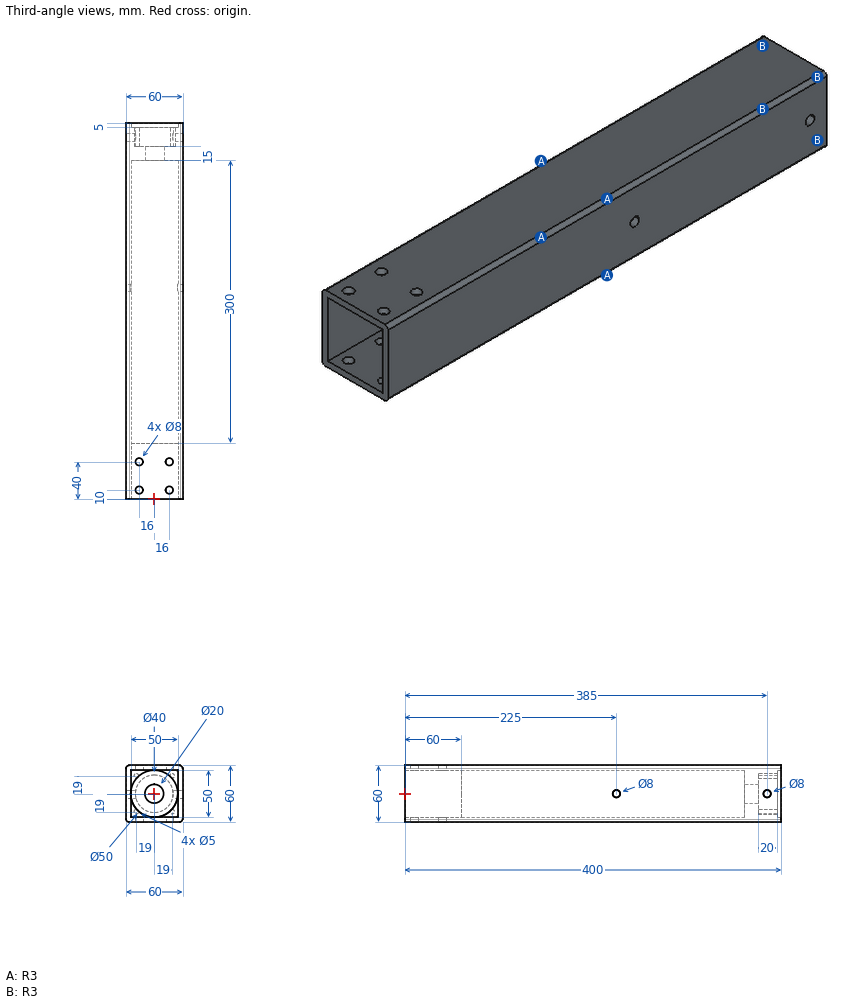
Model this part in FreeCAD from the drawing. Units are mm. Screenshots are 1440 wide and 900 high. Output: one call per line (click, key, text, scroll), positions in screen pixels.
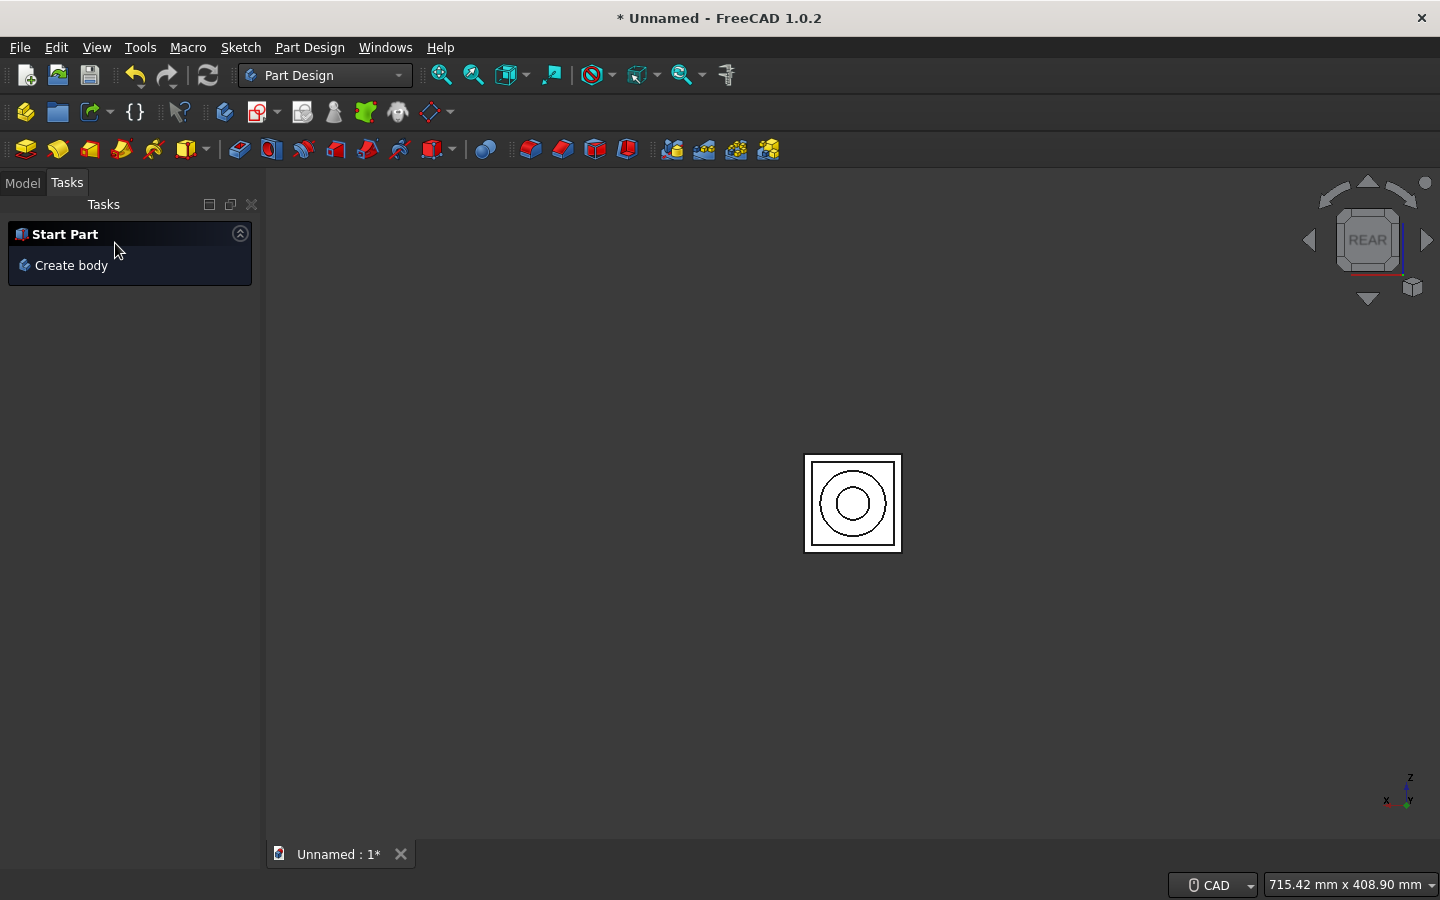
click(442, 76)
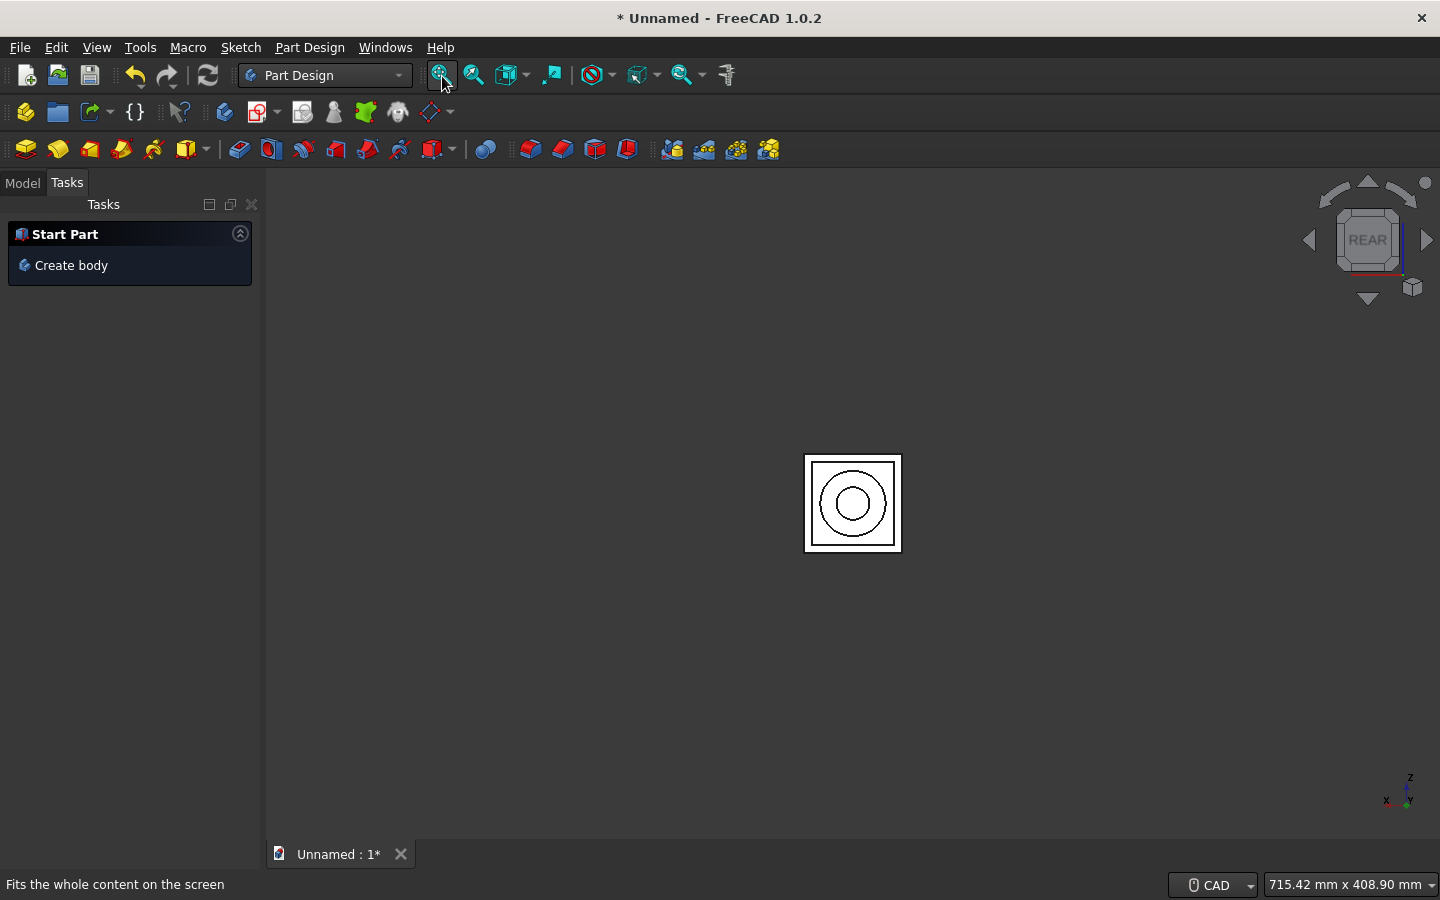
key(0)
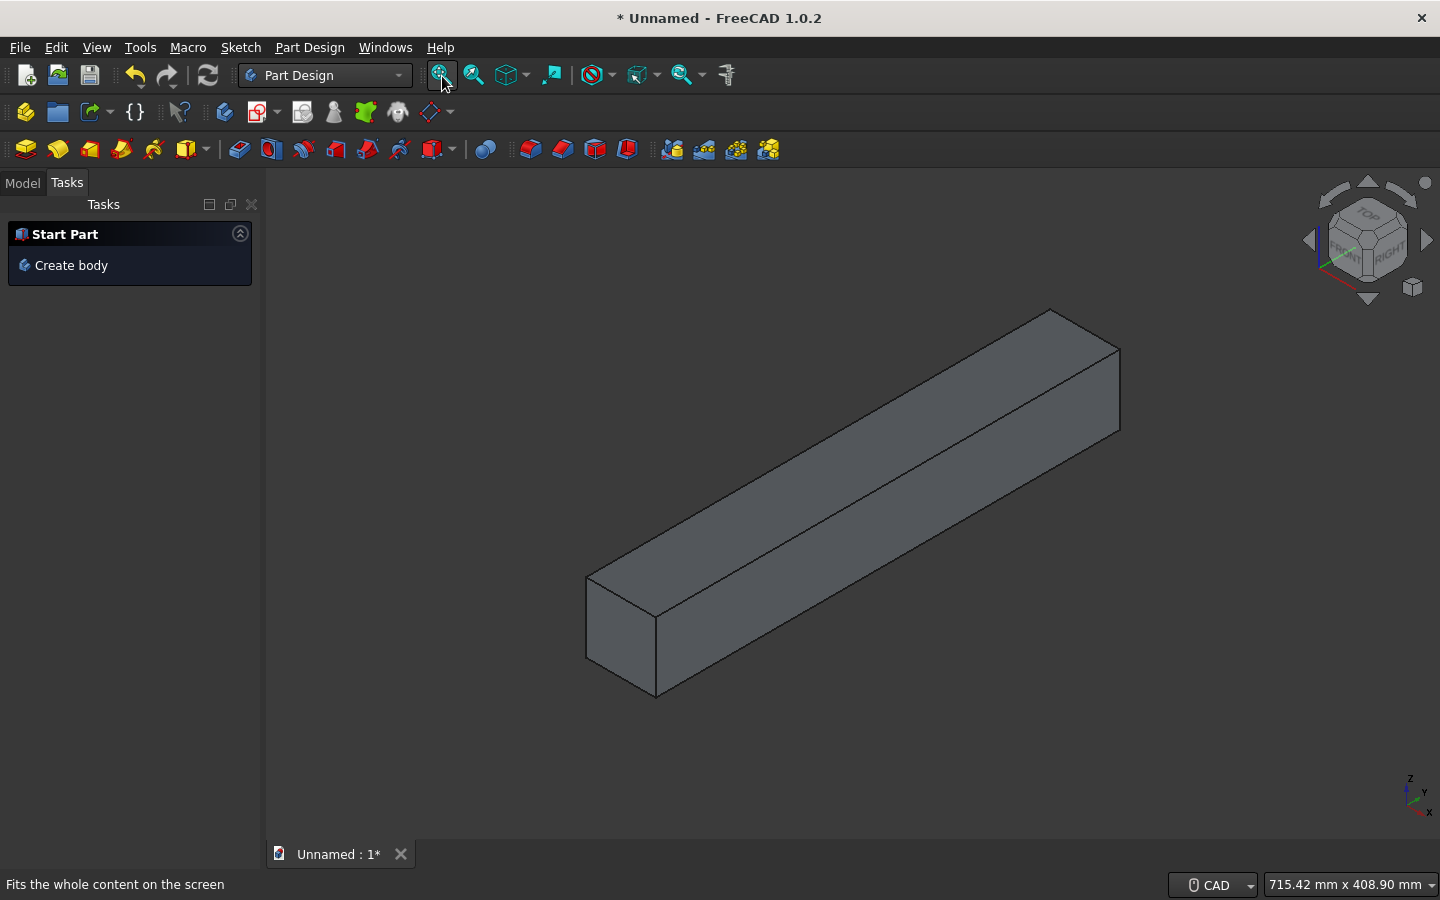
click(888, 482)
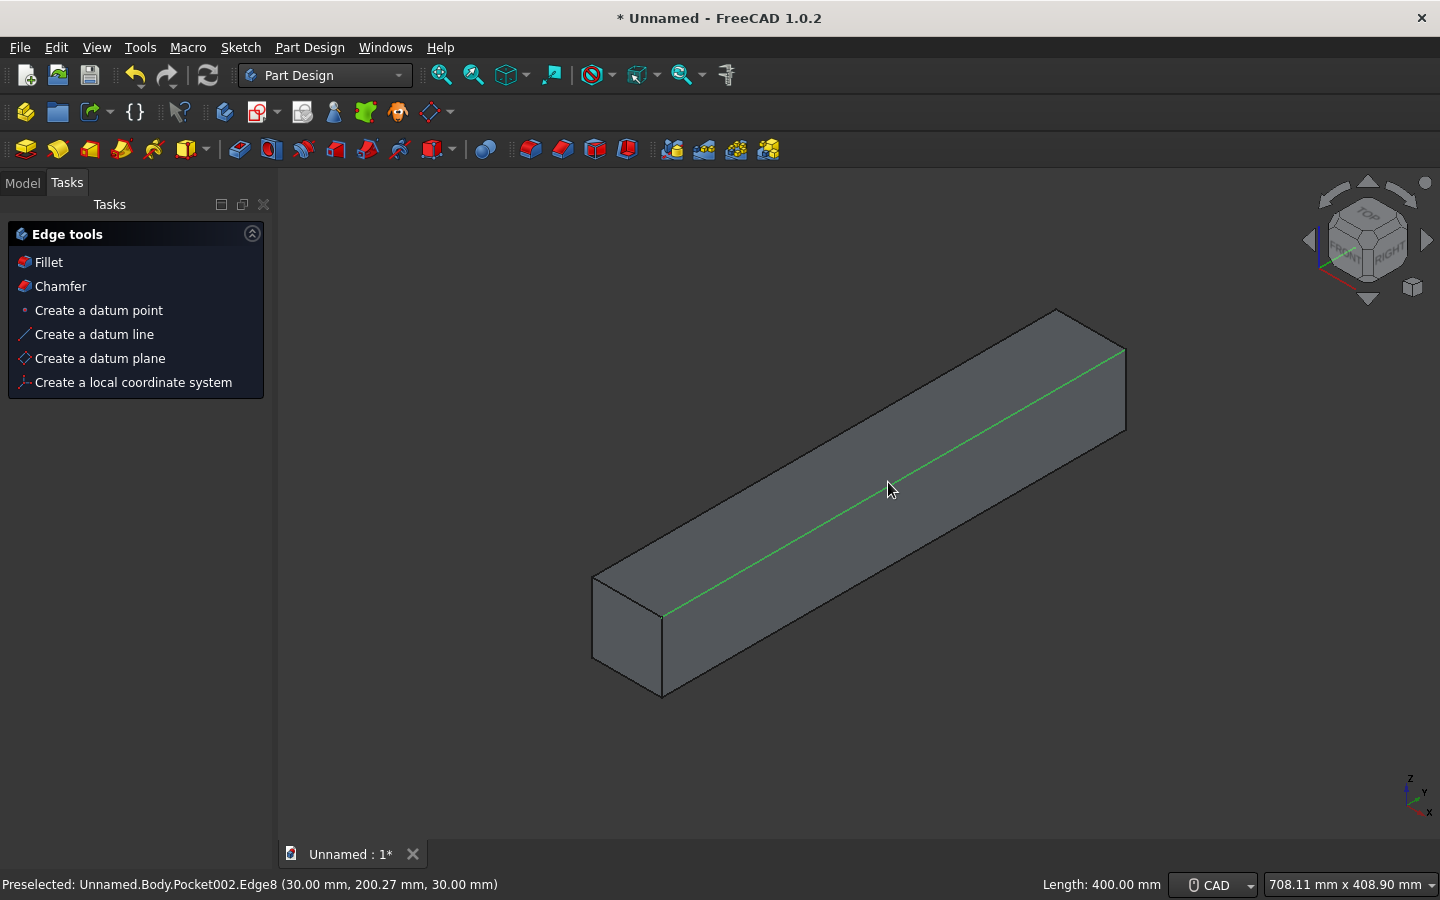
key(2)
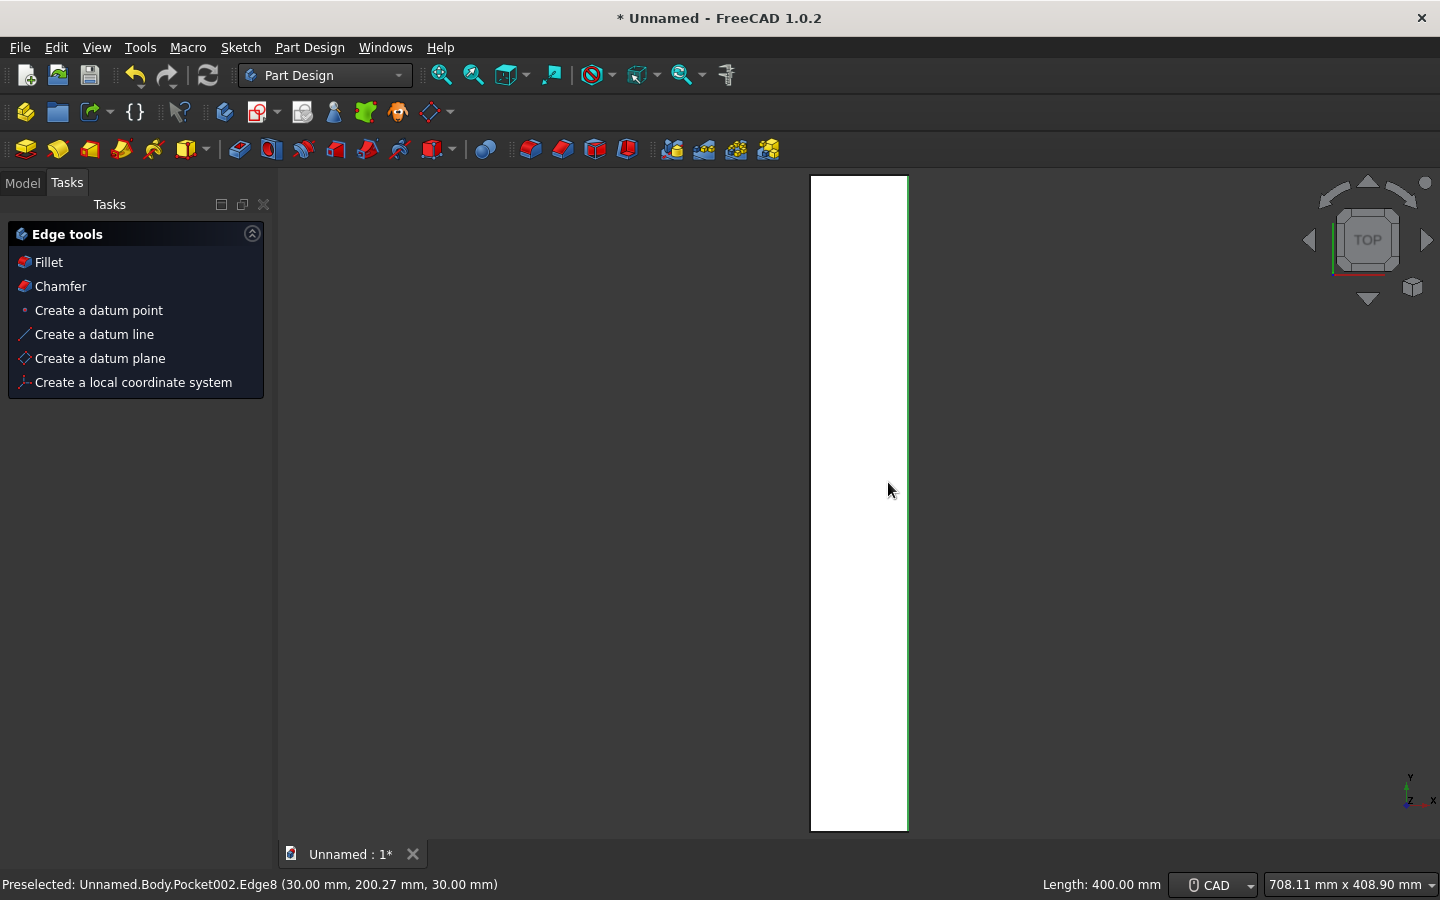
click(810, 503, ctrl)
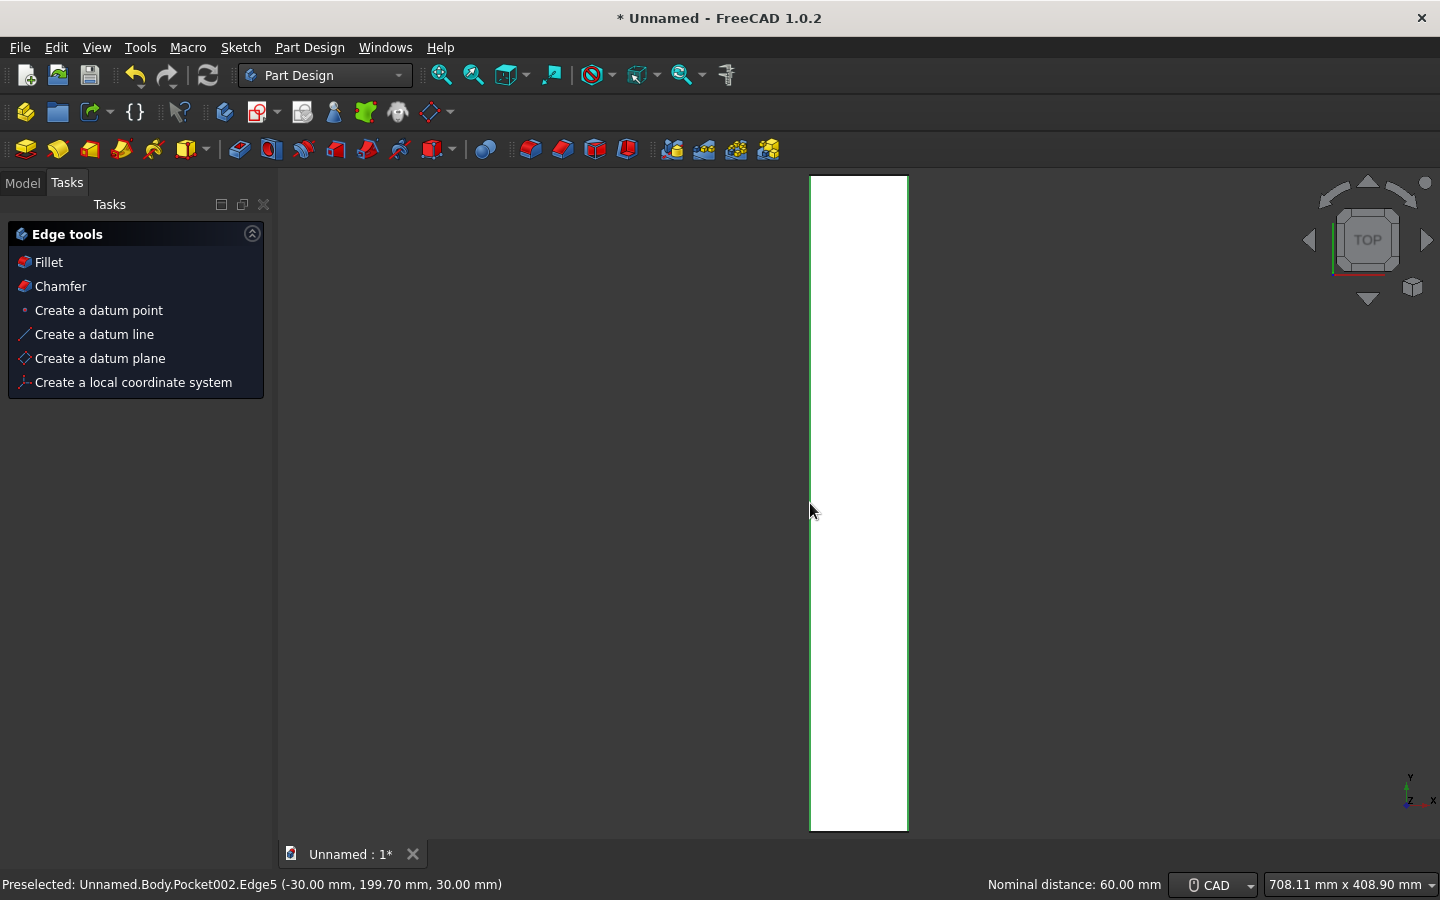
key(1)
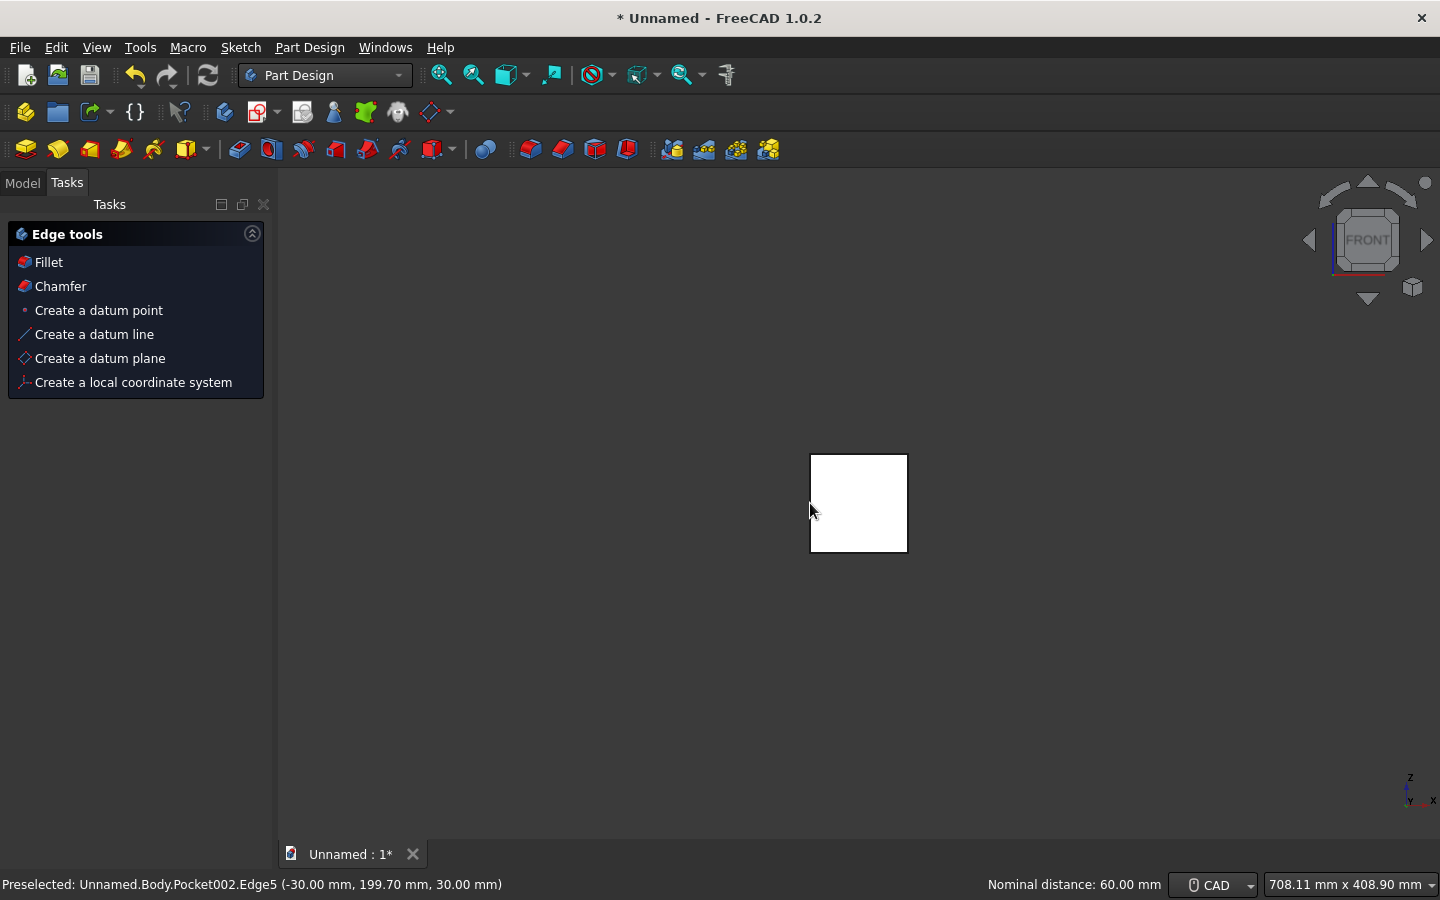
click(442, 76)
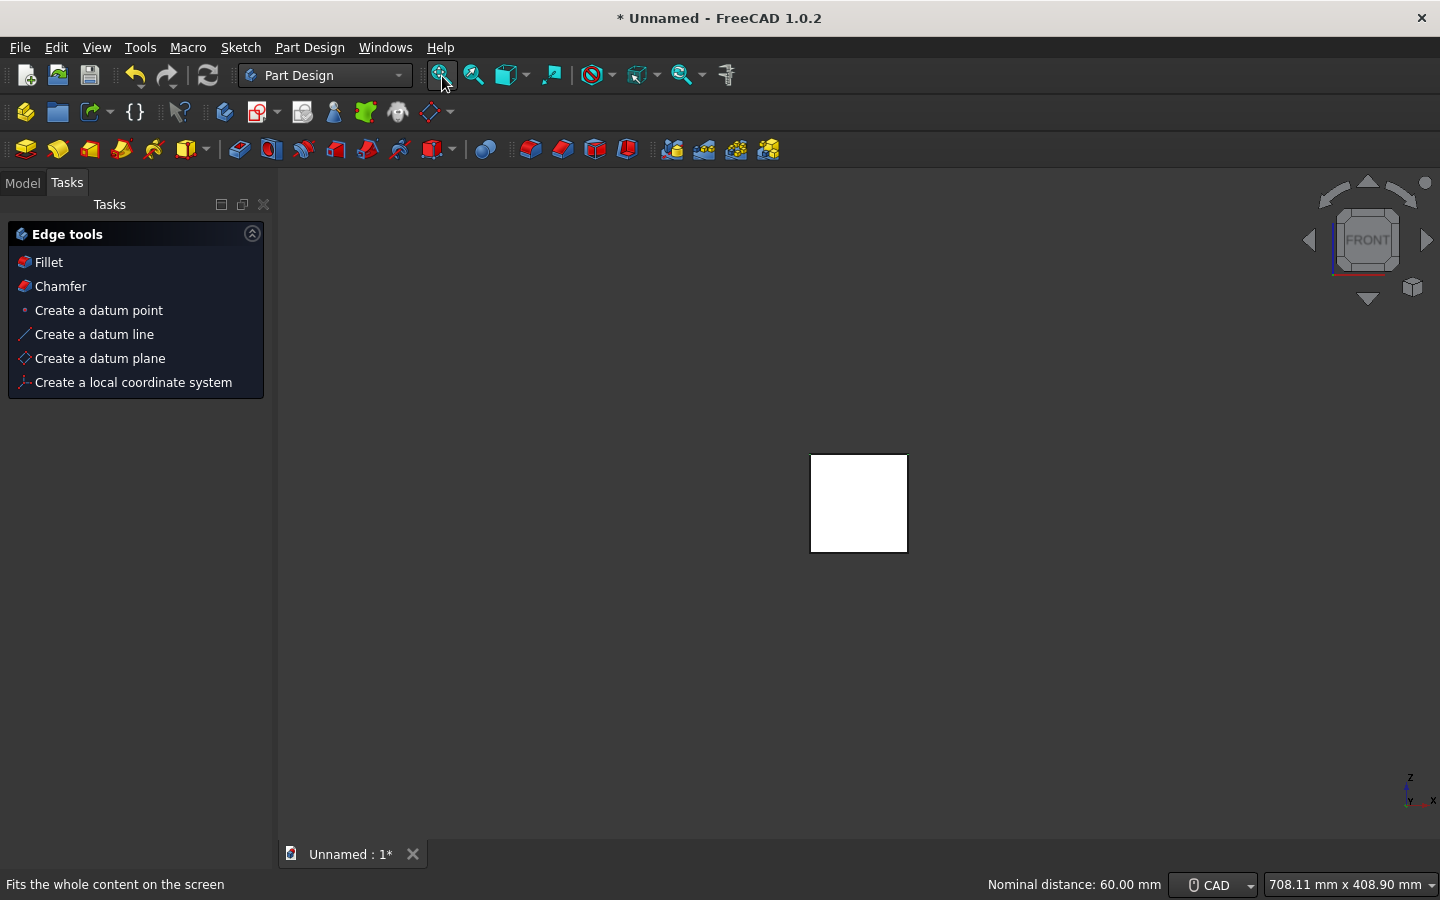
key(3)